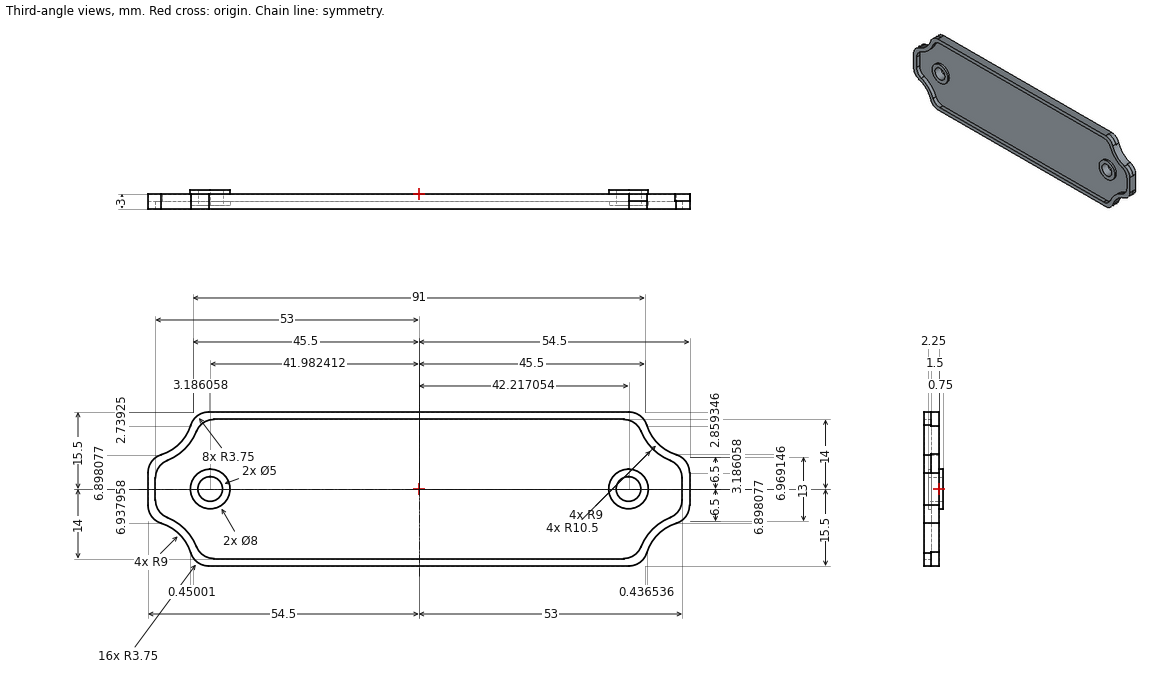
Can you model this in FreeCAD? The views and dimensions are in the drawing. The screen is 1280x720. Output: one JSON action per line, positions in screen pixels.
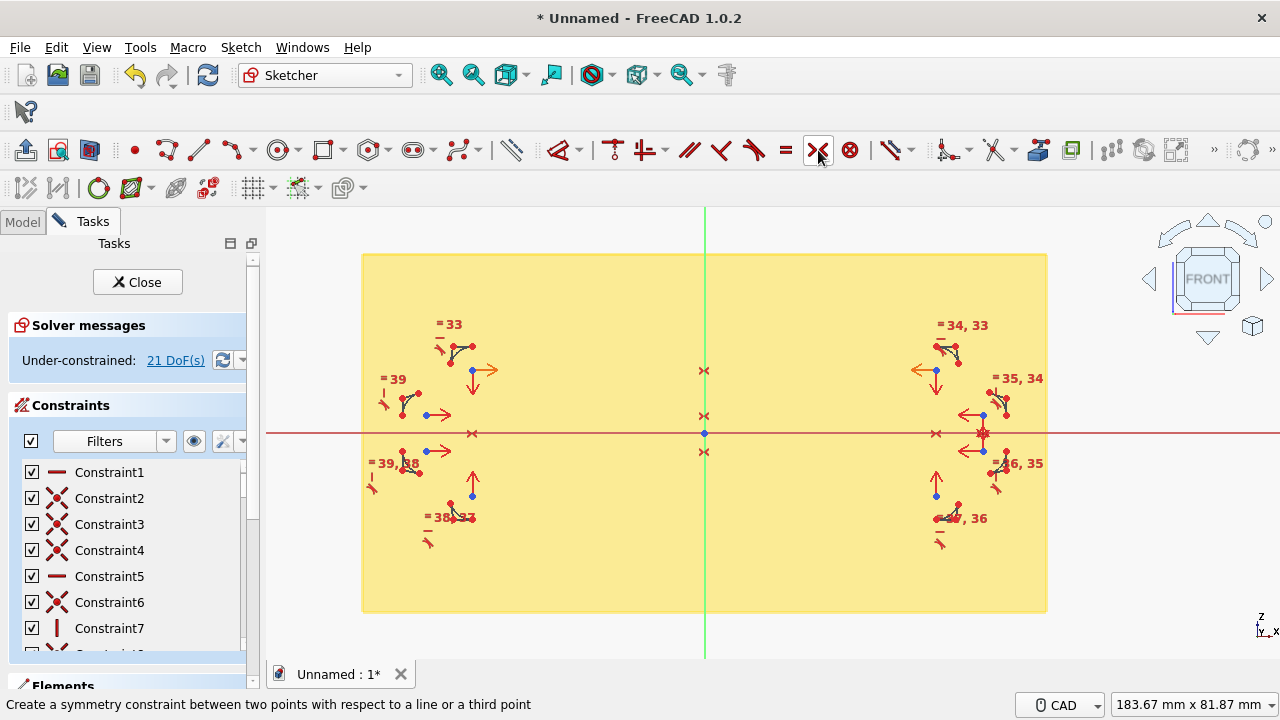
{"action": "left_click", "coordinate": [558, 150]}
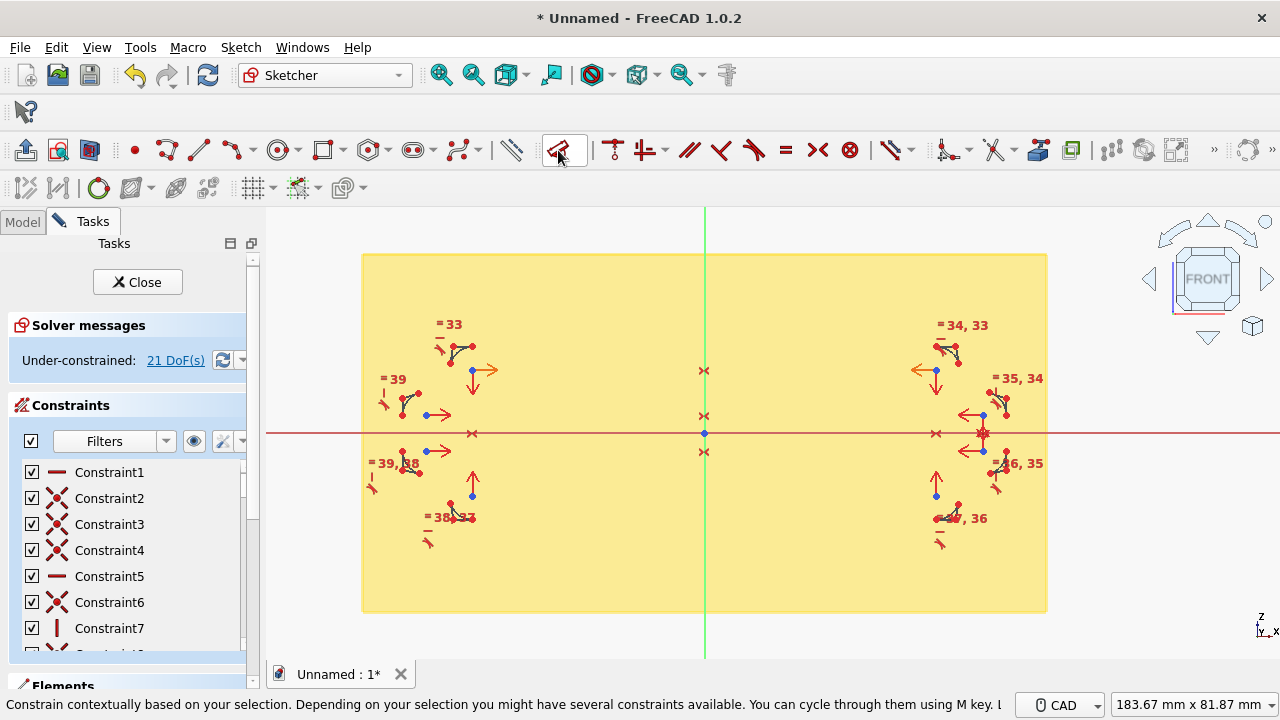
{"action": "scroll", "coordinate": [459, 351], "scroll_direction": "up", "scroll_amount": 6}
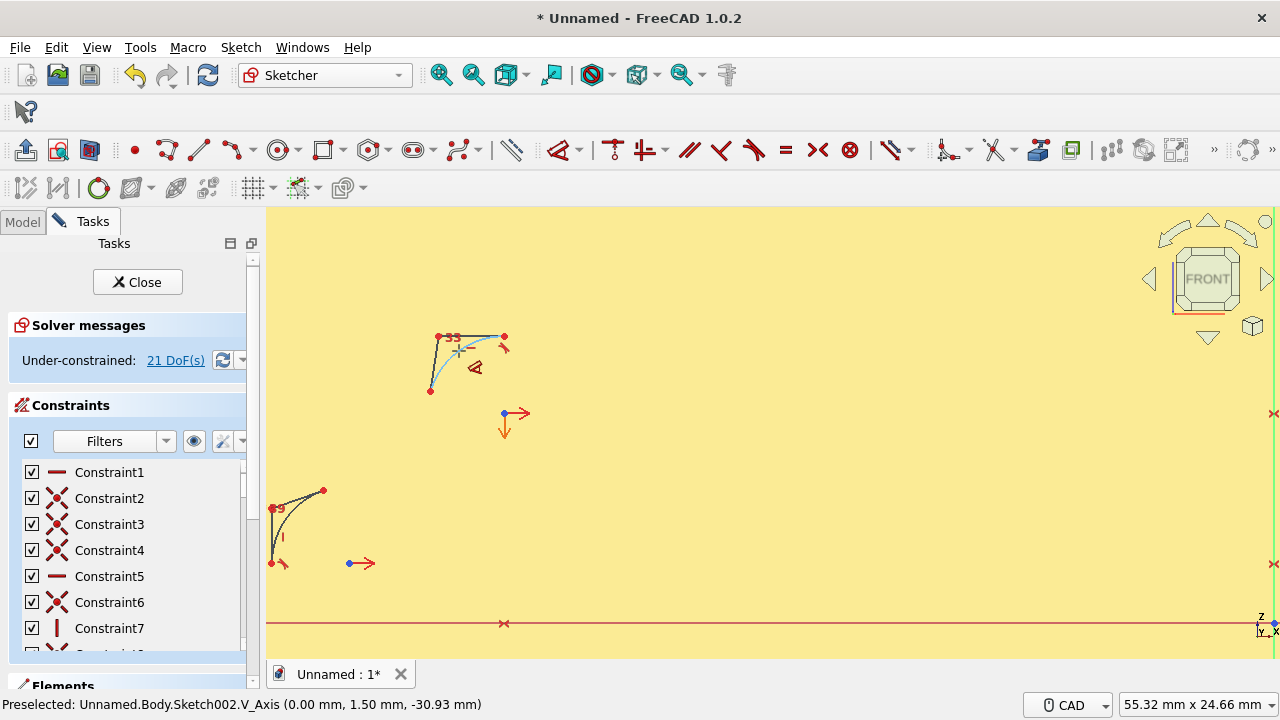
{"action": "left_click", "coordinate": [458, 352]}
{"action": "left_click", "coordinate": [488, 306]}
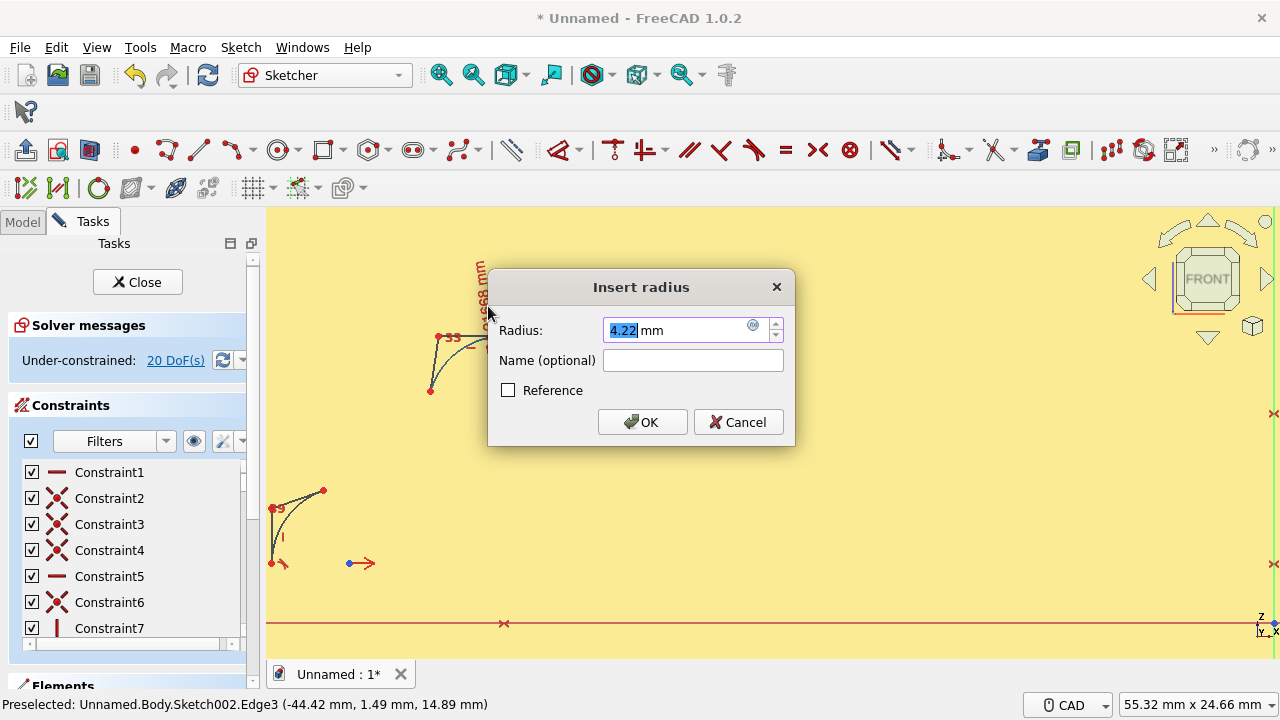
{"action": "type", "text": "3.75"}
{"action": "key", "text": "Return"}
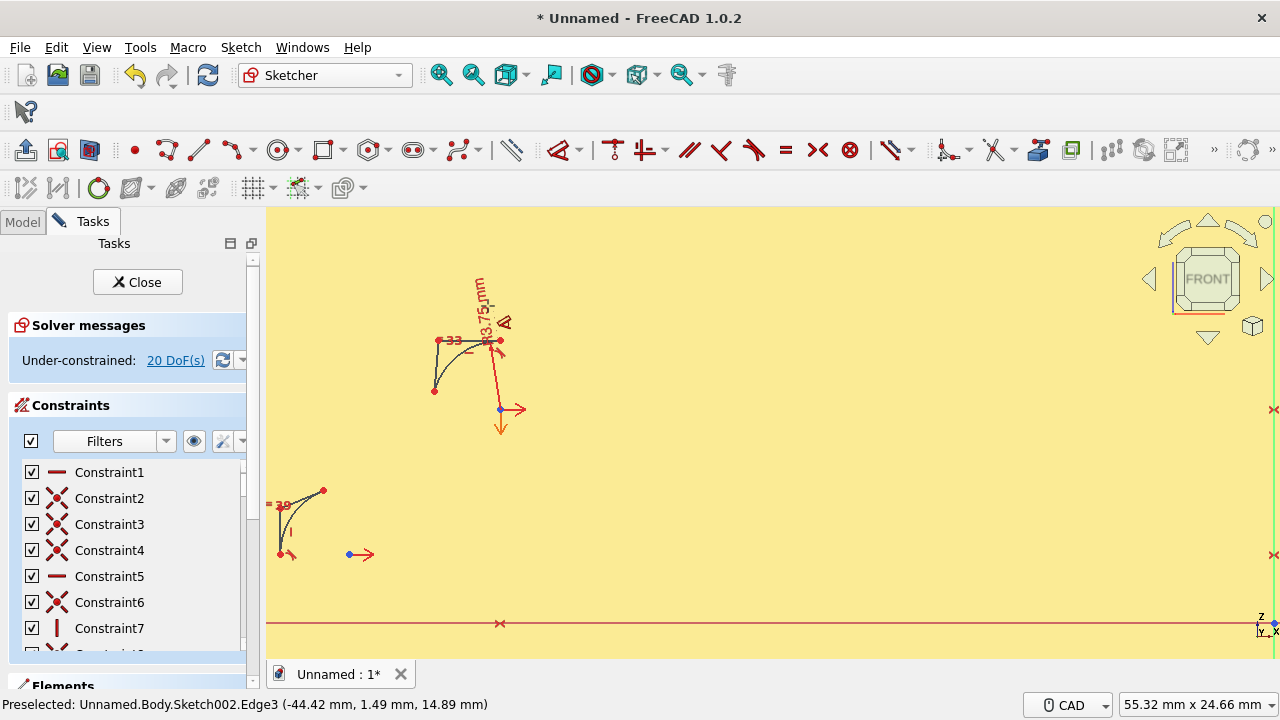
{"action": "scroll", "coordinate": [459, 351], "scroll_direction": "down", "scroll_amount": 6}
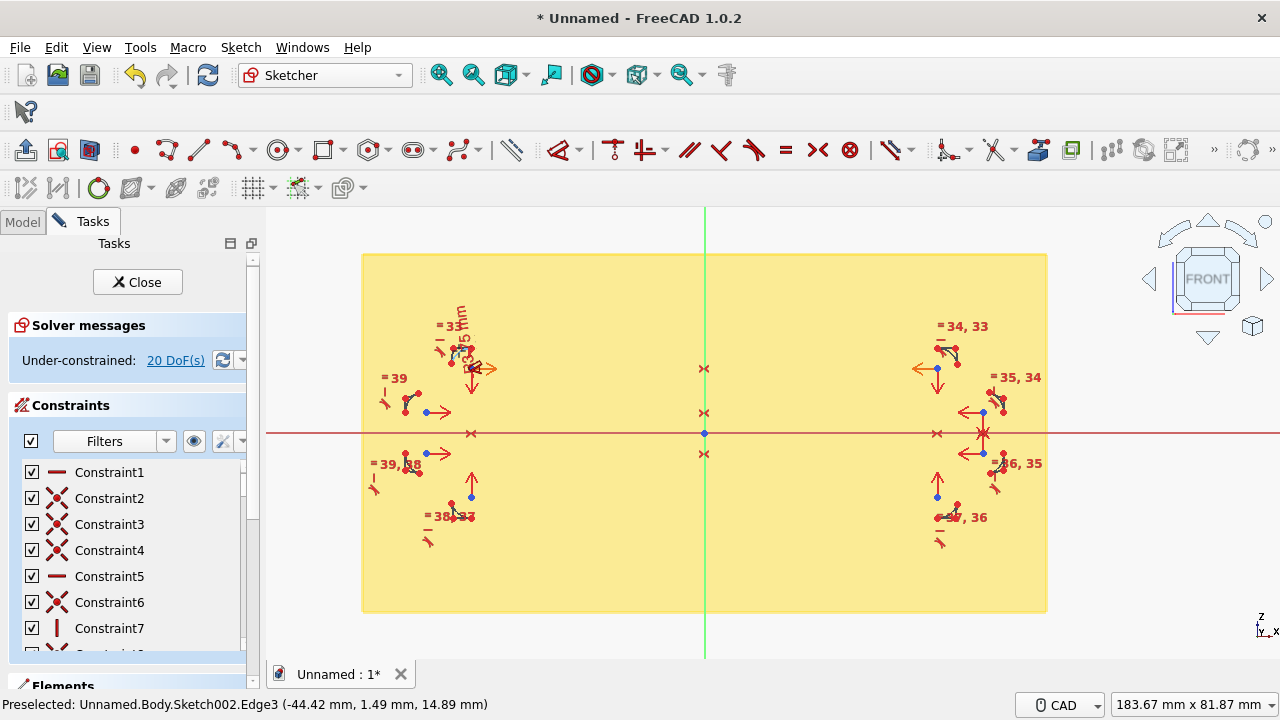
{"action": "left_click", "coordinate": [1004, 399]}
{"action": "left_click", "coordinate": [1038, 416]}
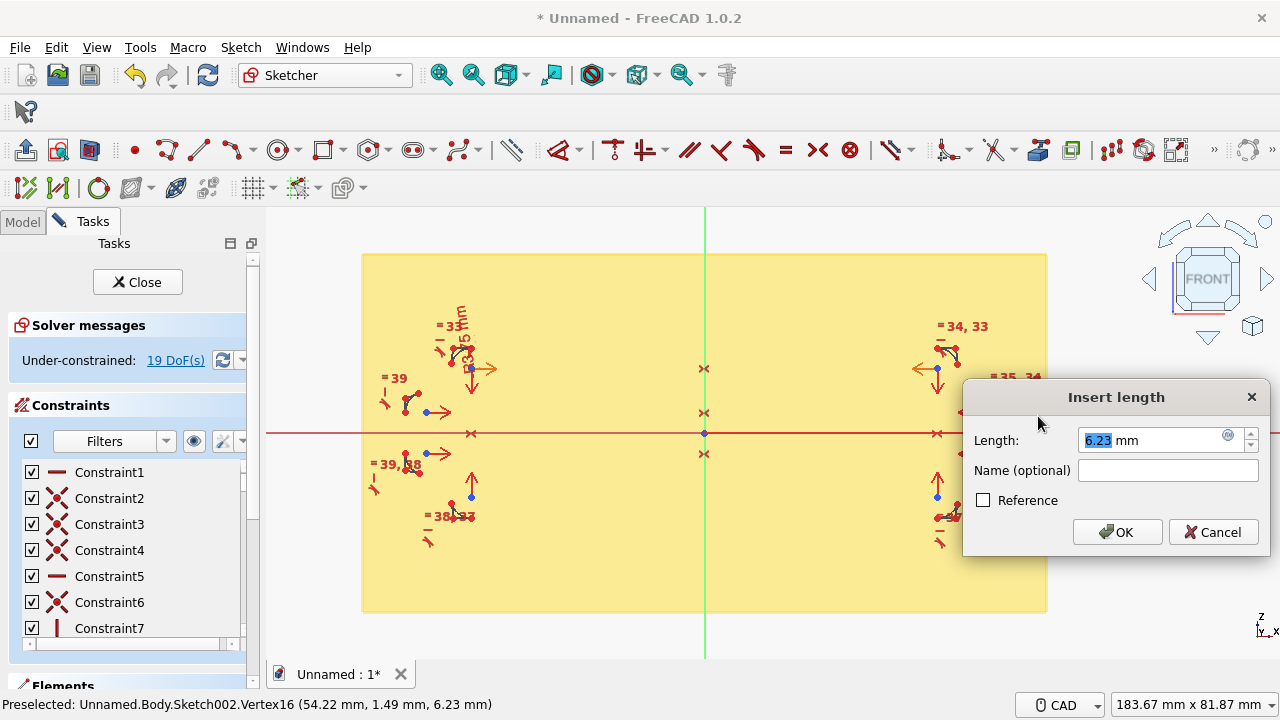
{"action": "type", "text": "6.5"}
{"action": "key", "text": "Return"}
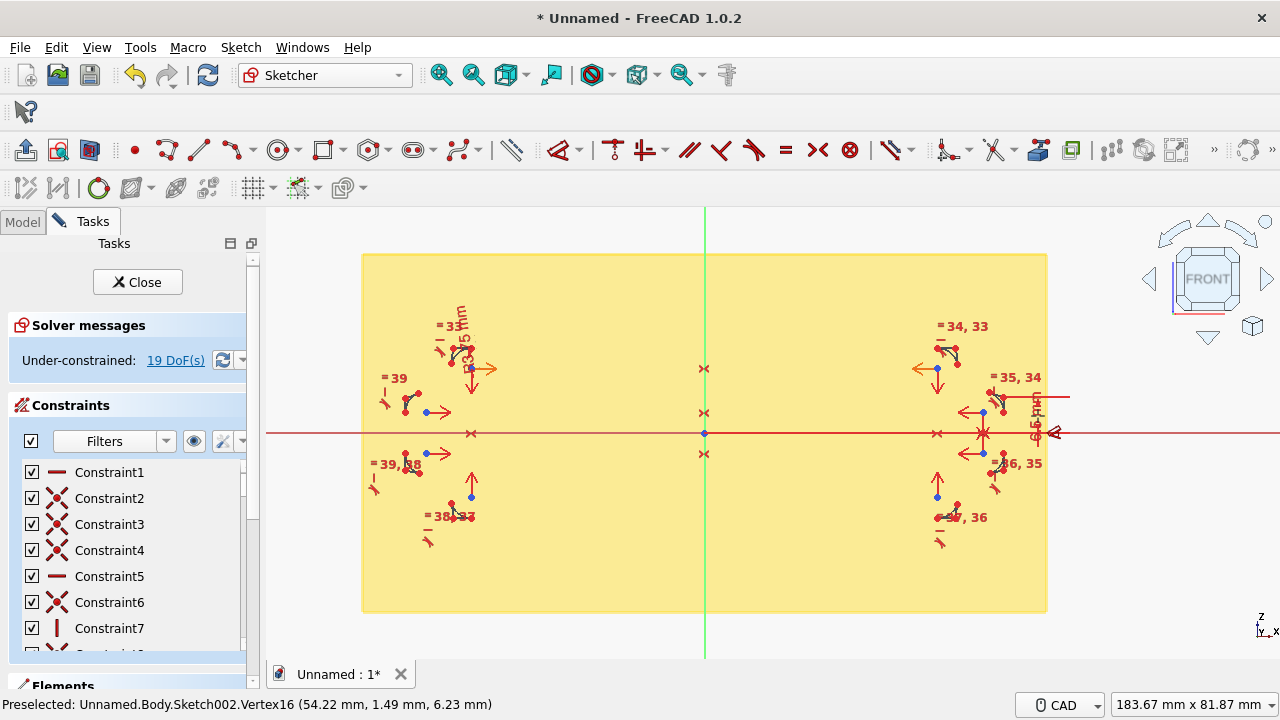
{"action": "left_click", "coordinate": [1004, 470]}
{"action": "left_click", "coordinate": [1038, 452]}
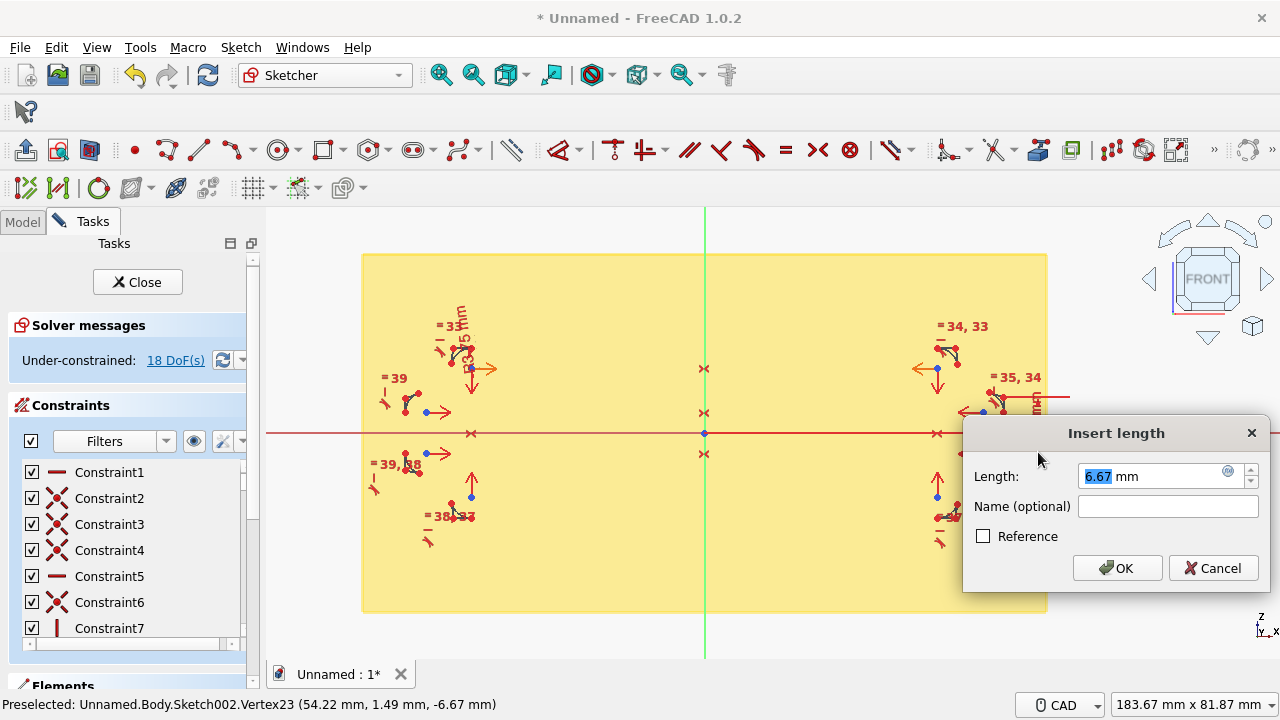
{"action": "type", "text": "6.5"}
{"action": "key", "text": "Return"}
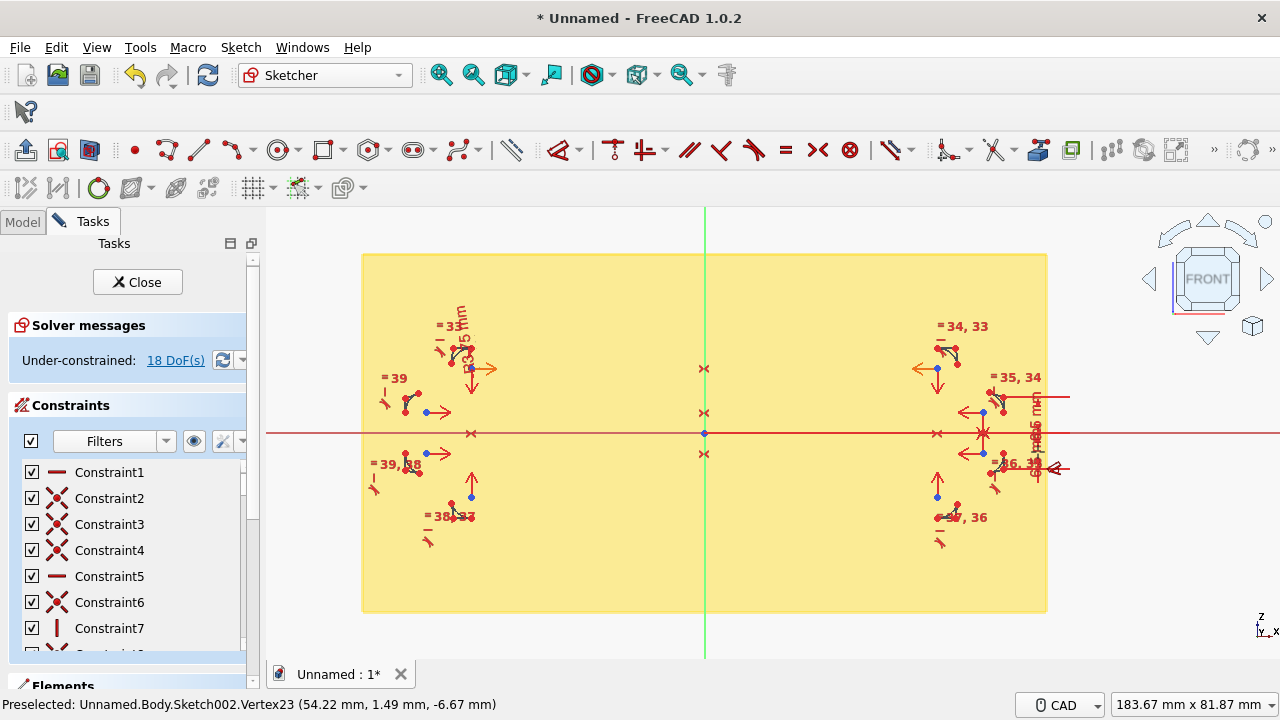
{"action": "left_click", "coordinate": [405, 470]}
{"action": "left_click", "coordinate": [371, 452]}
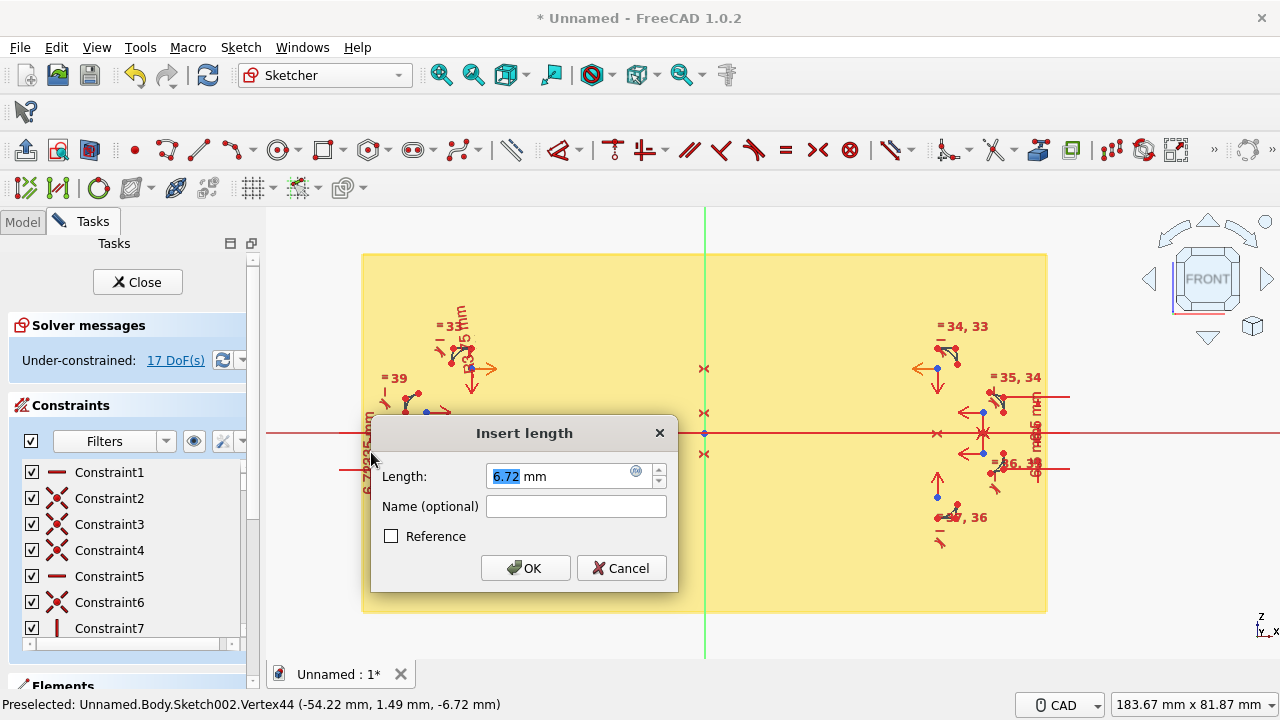
{"action": "type", "text": "6.5"}
{"action": "key", "text": "Return"}